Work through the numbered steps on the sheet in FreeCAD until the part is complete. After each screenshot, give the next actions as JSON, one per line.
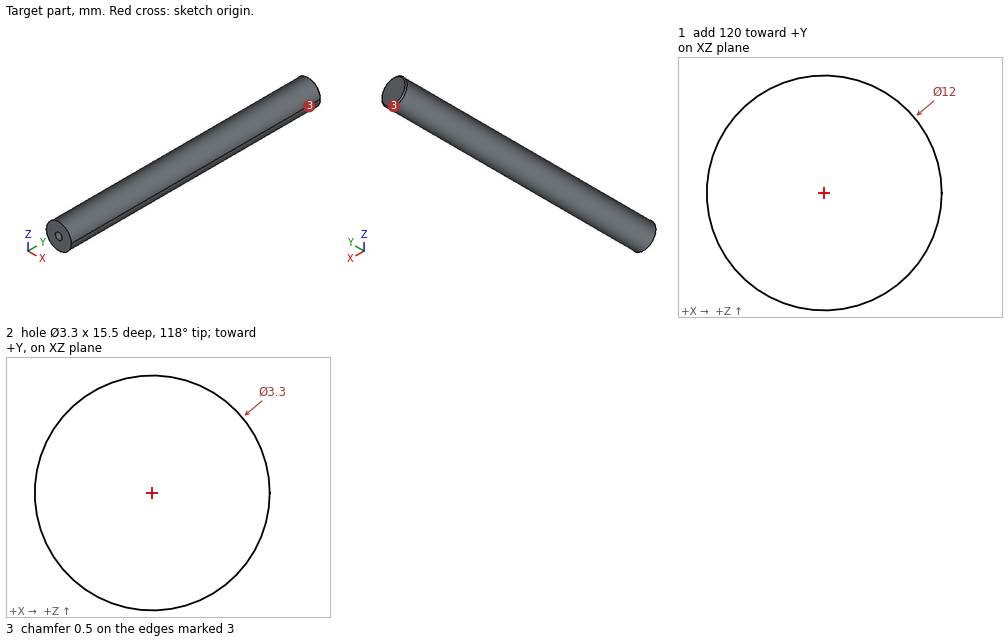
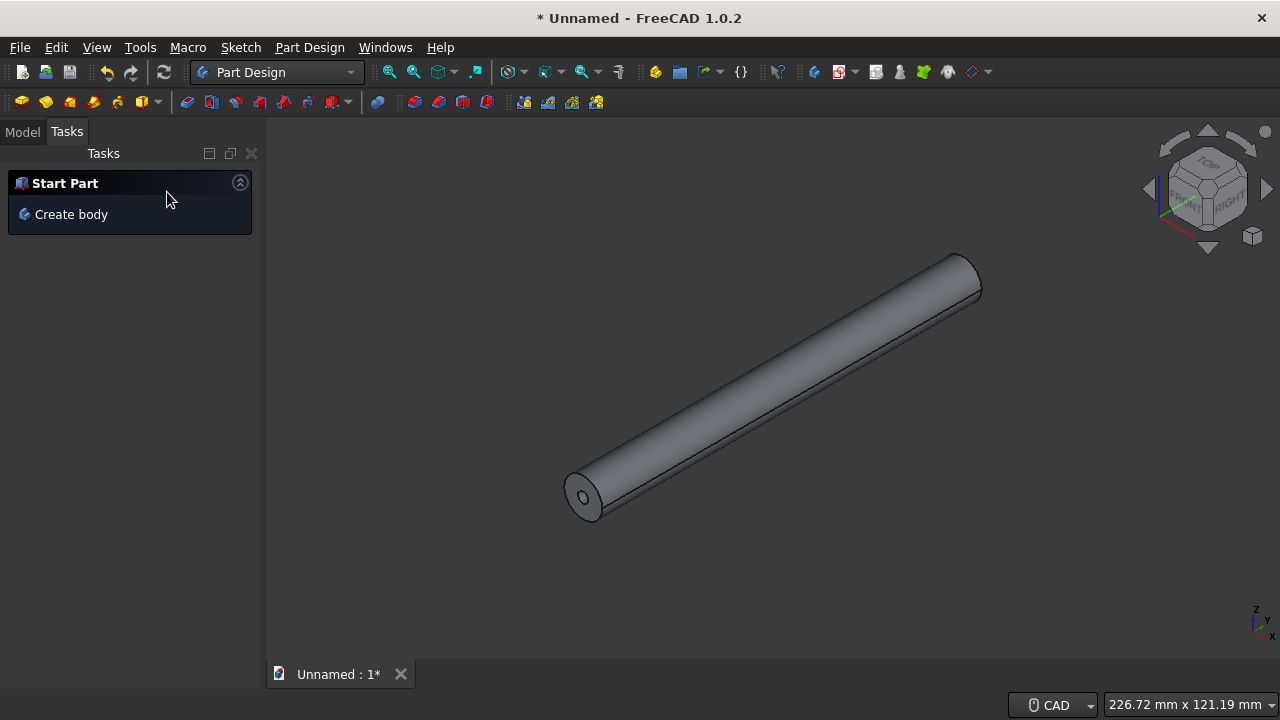
{"action": "key", "text": "2"}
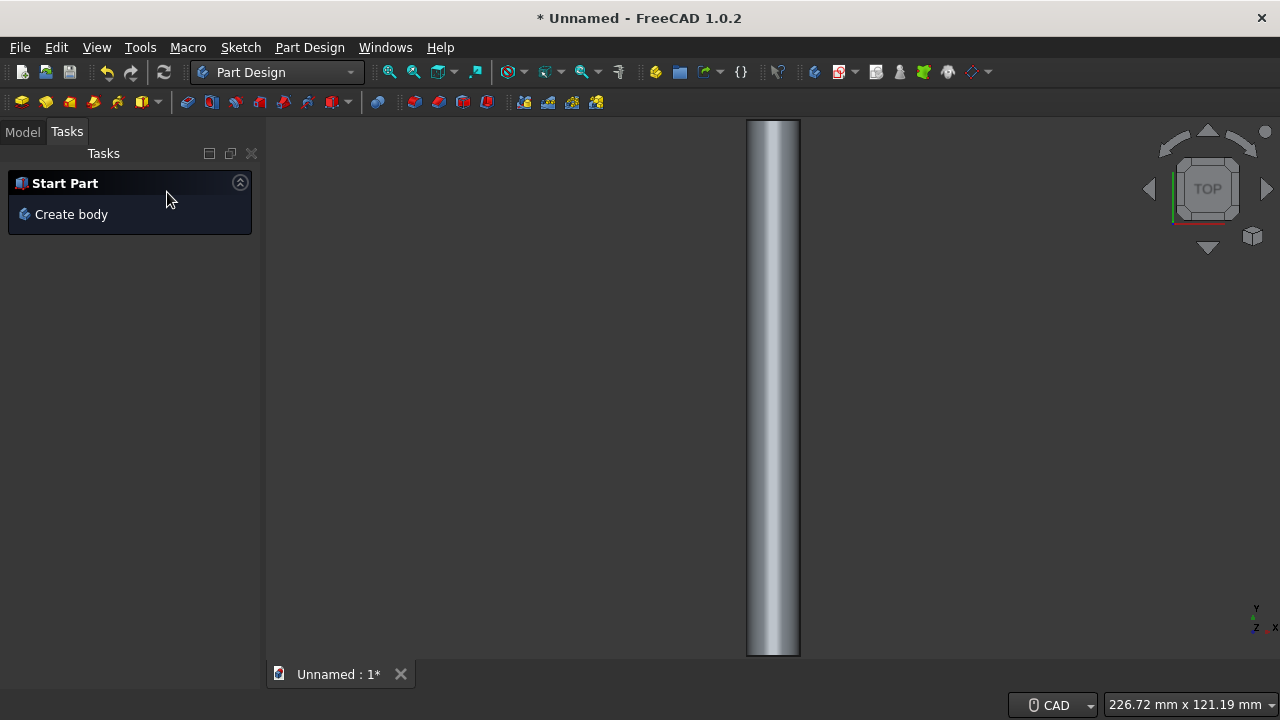
{"action": "key", "text": "1"}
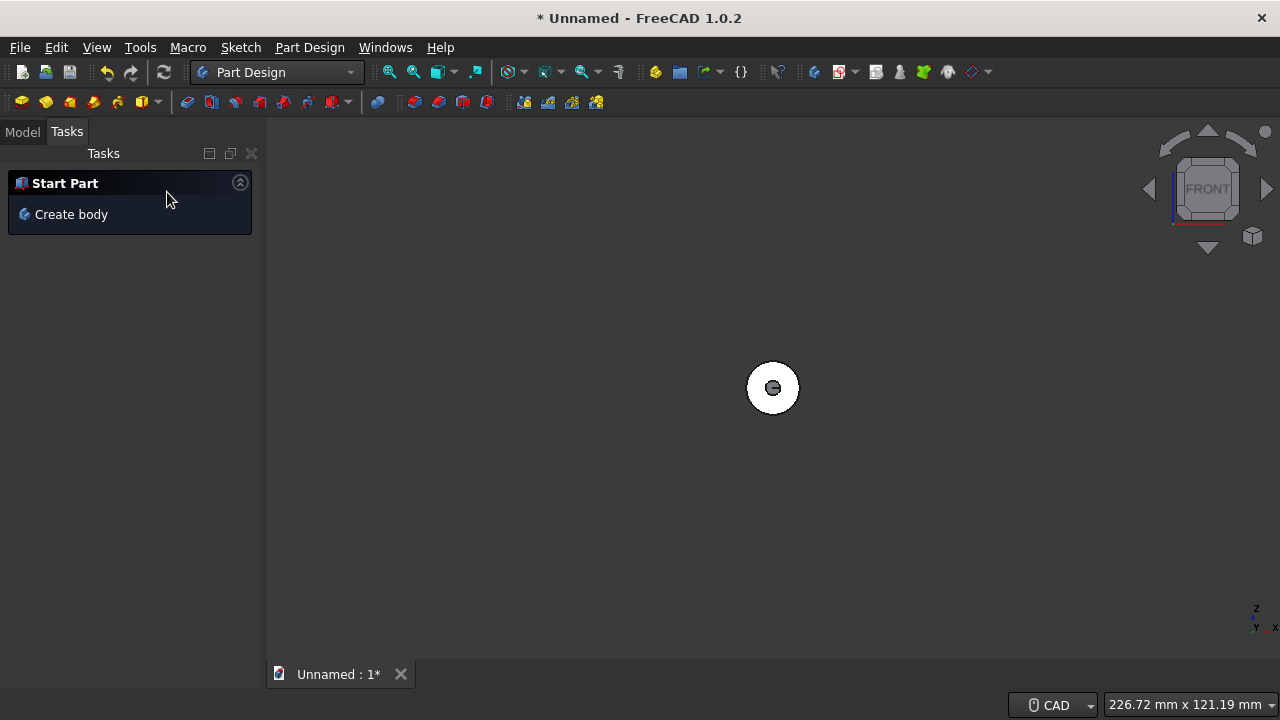
{"action": "left_click", "coordinate": [390, 72]}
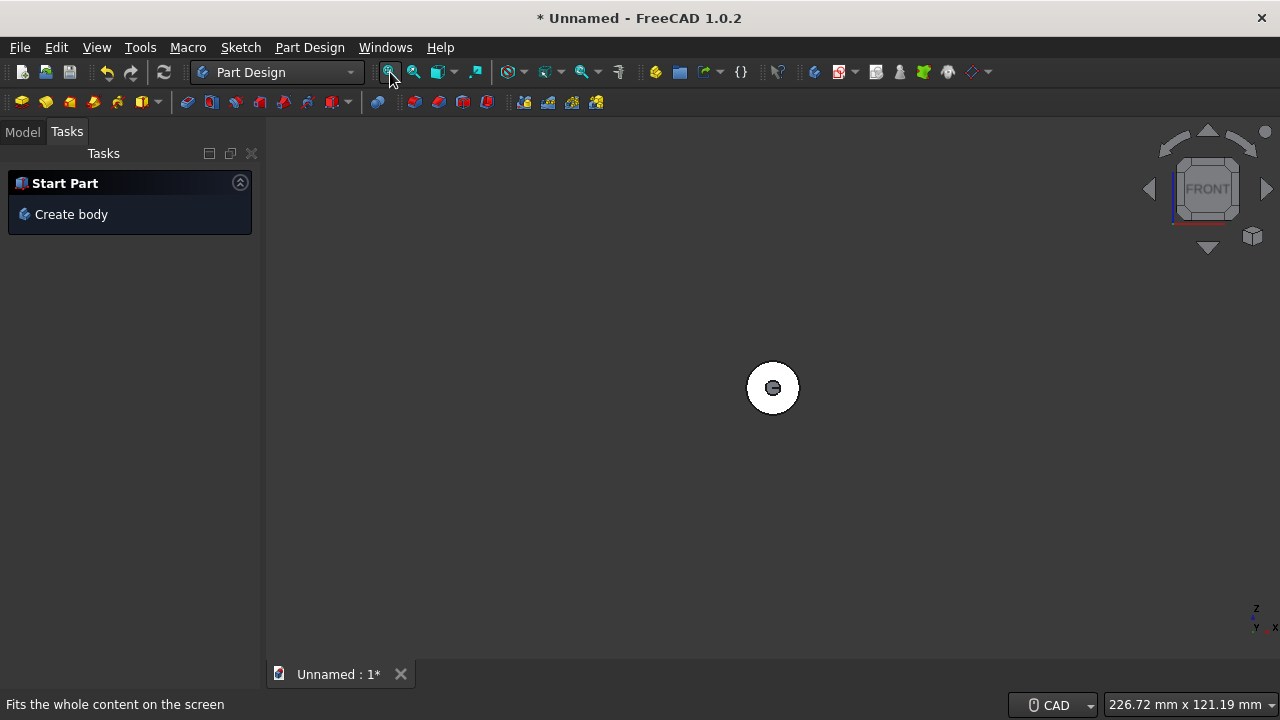
{"action": "key", "text": "3"}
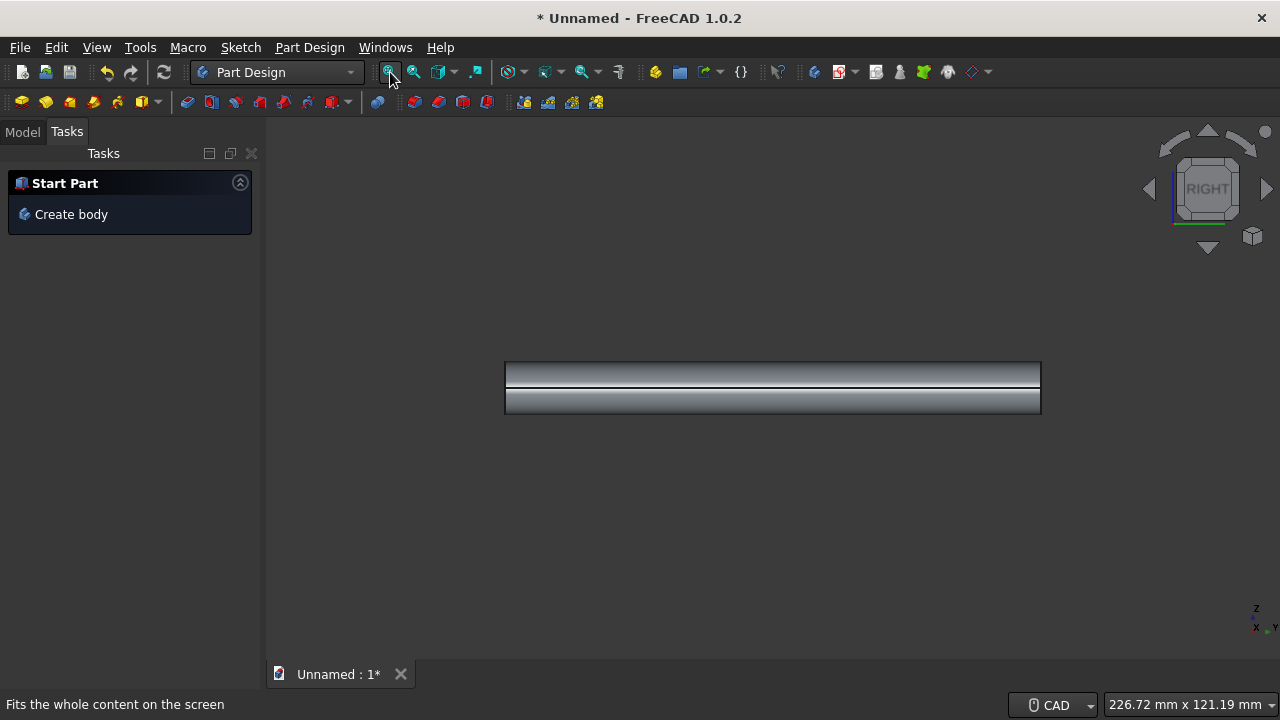
{"action": "left_click", "coordinate": [1041, 371]}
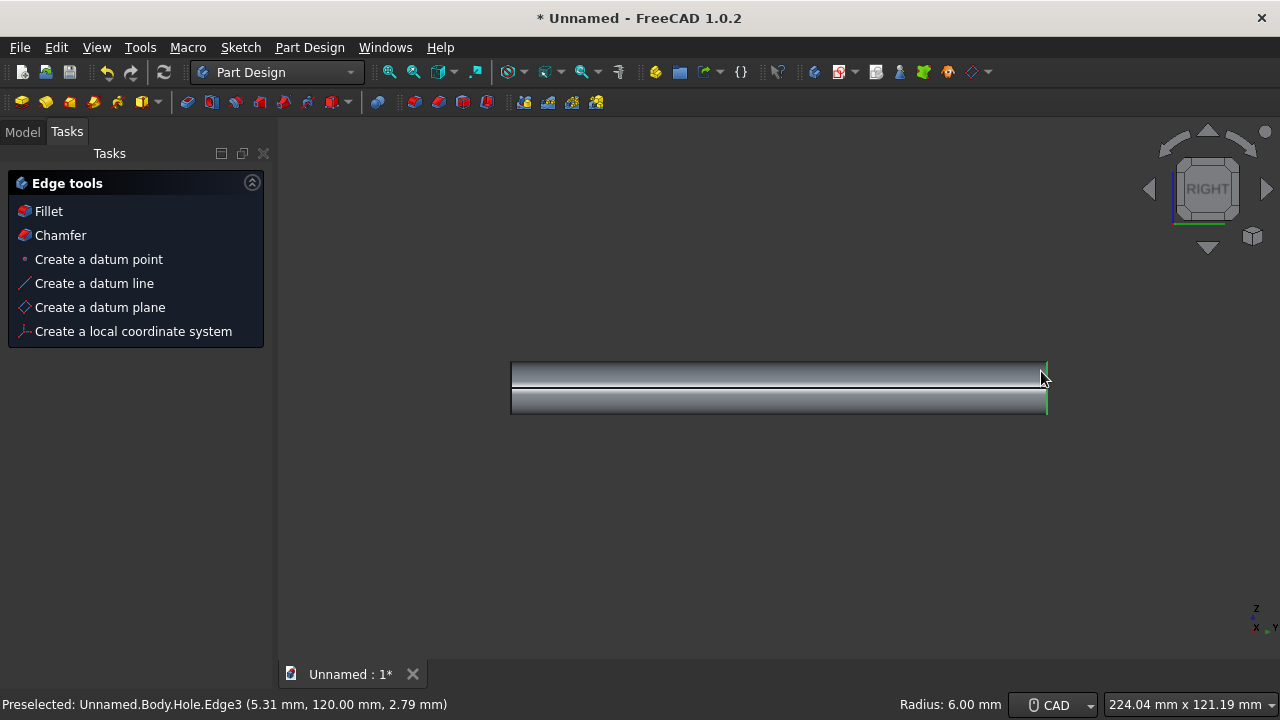
{"action": "left_click", "coordinate": [440, 102]}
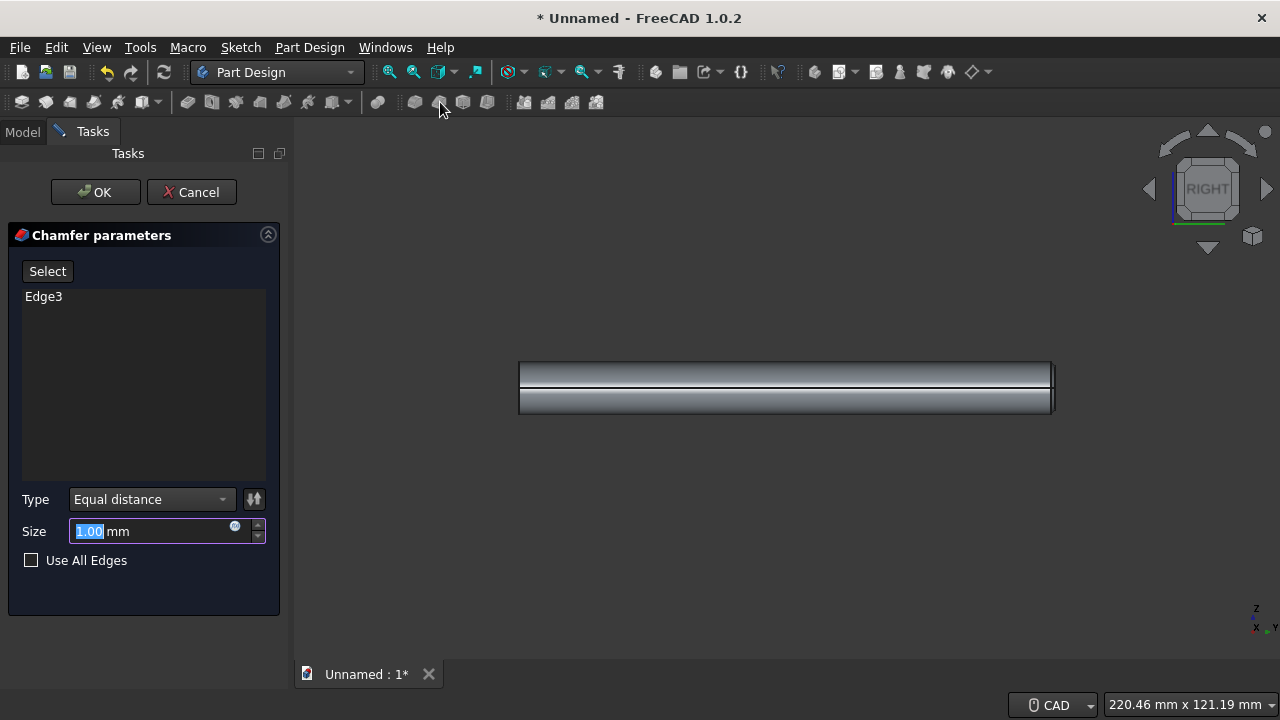
{"action": "type", "text": "0.5"}
{"action": "key", "text": "Tab"}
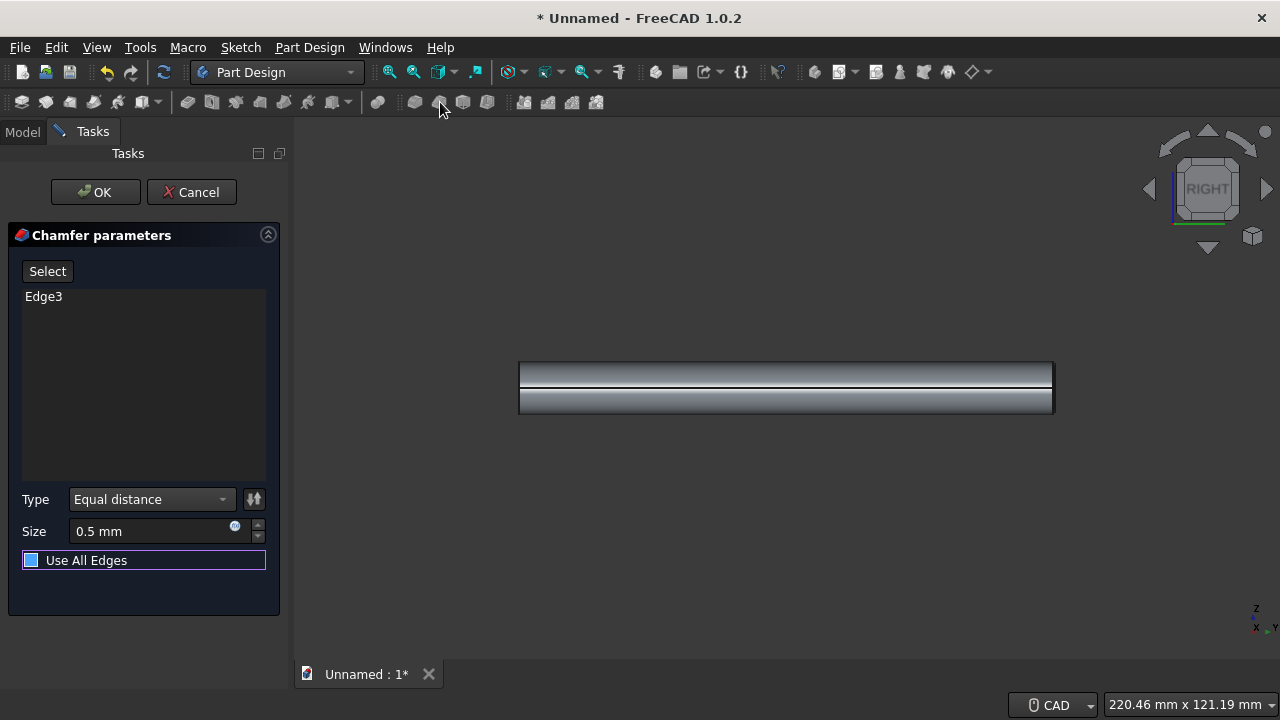
{"action": "left_click", "coordinate": [96, 192]}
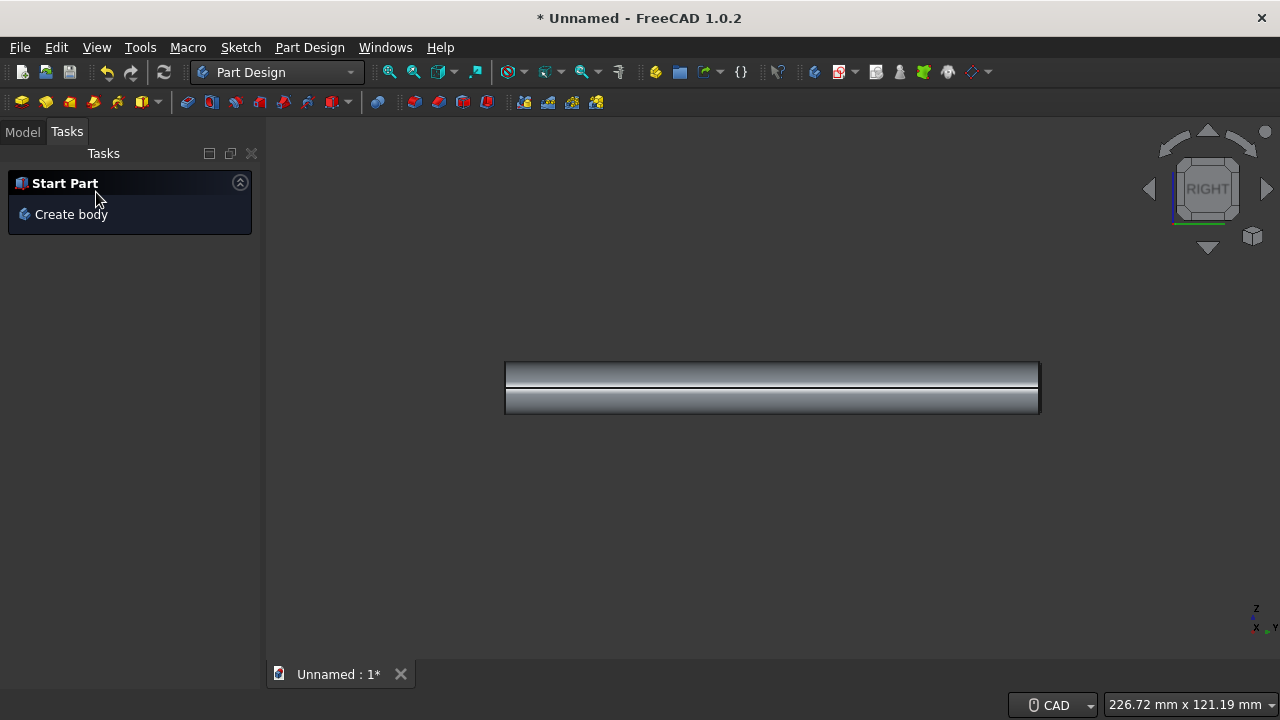
{"action": "key", "text": "0"}